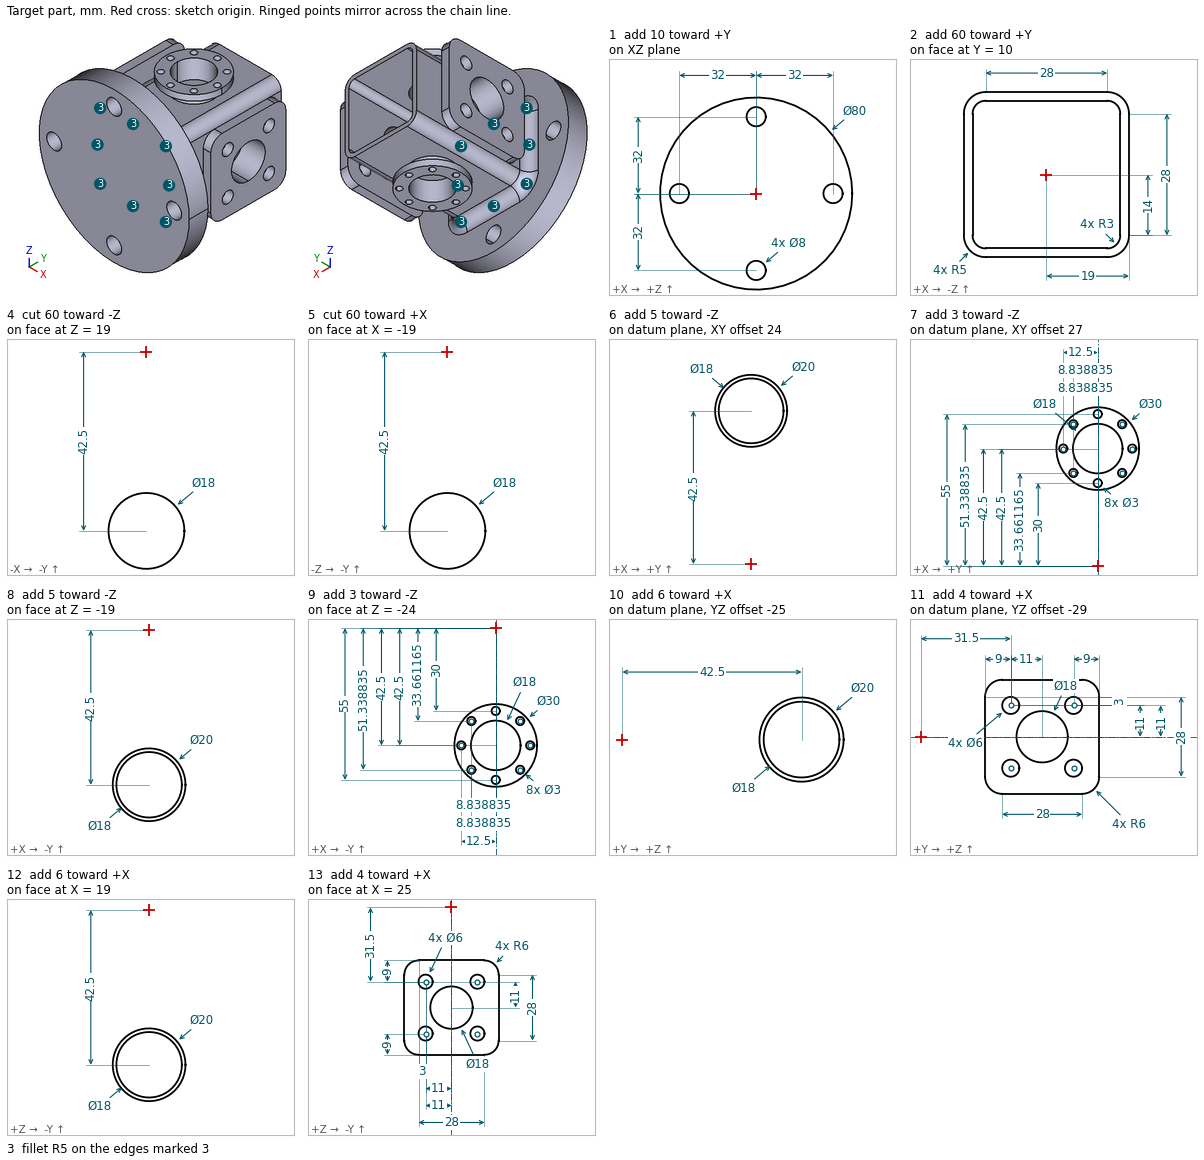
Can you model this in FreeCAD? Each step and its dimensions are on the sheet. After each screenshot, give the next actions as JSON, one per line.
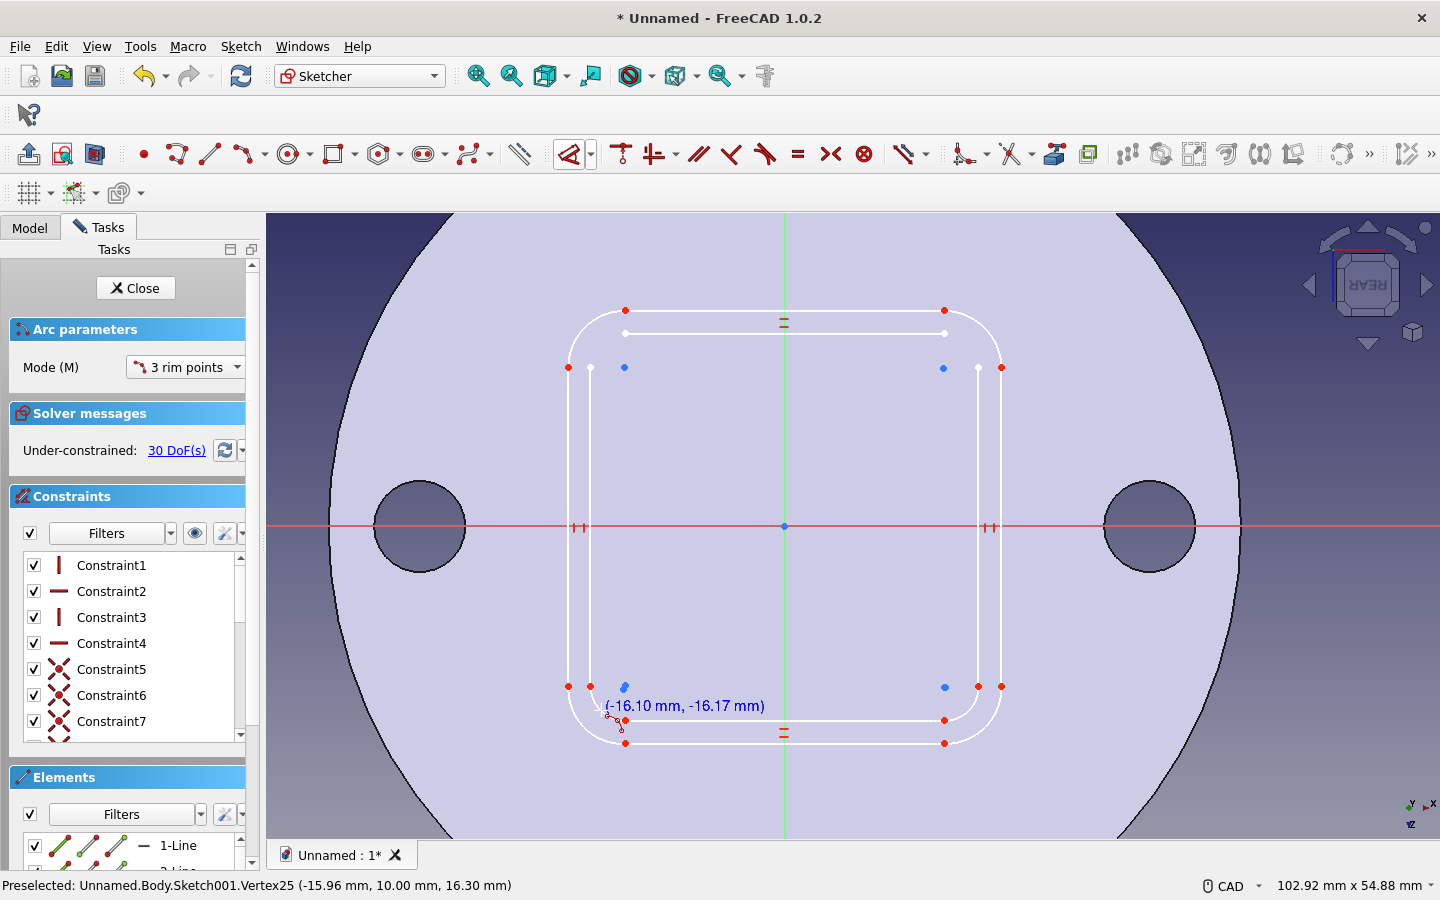
{"action": "left_click", "coordinate": [590, 368]}
{"action": "left_click", "coordinate": [625, 334]}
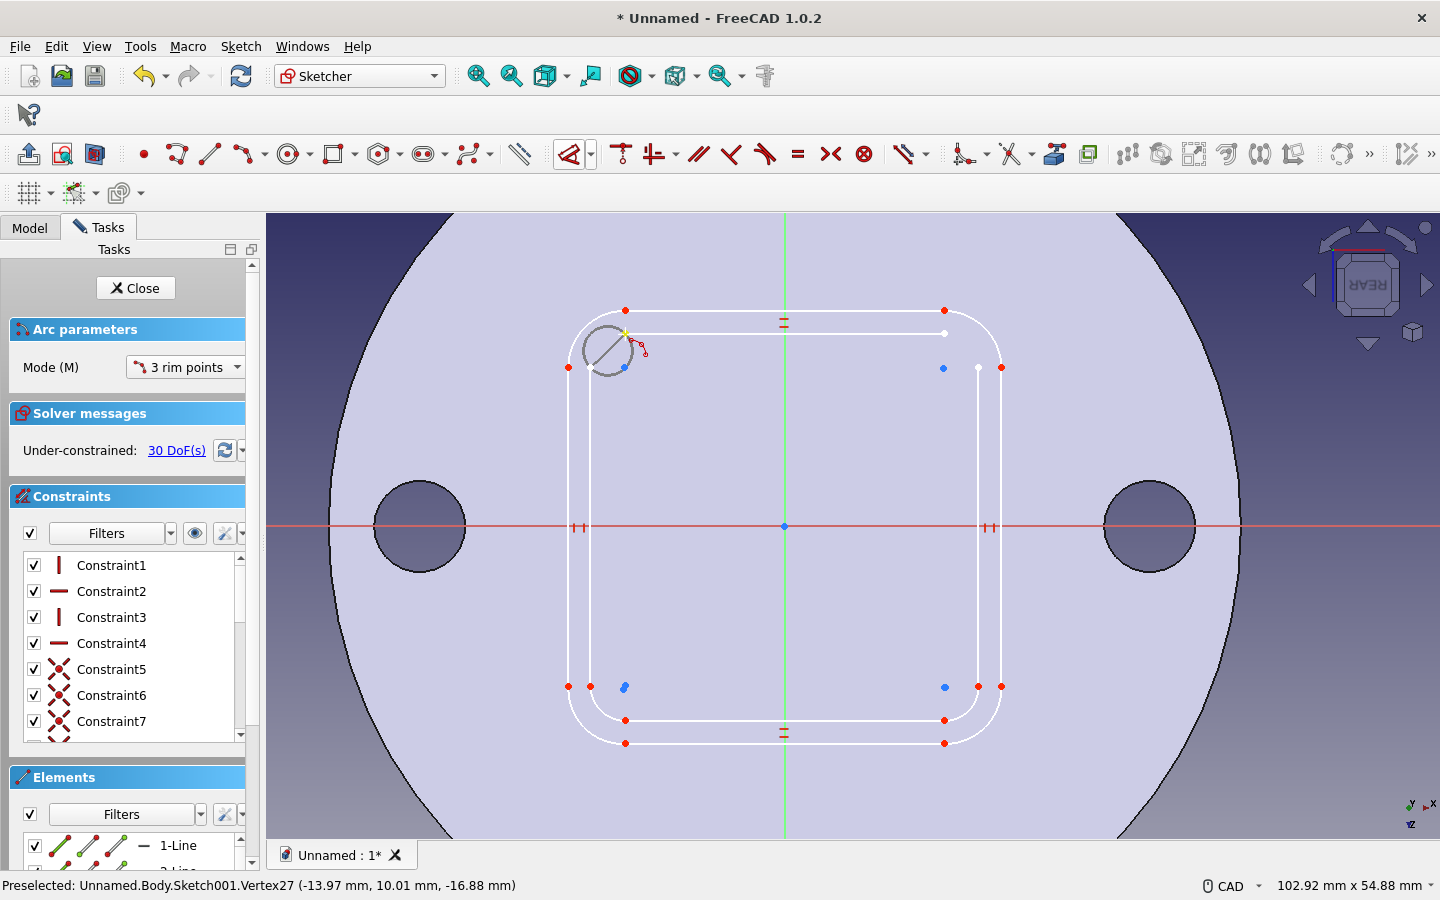
{"action": "scroll", "coordinate": [601, 343], "scroll_direction": "up", "scroll_amount": 3}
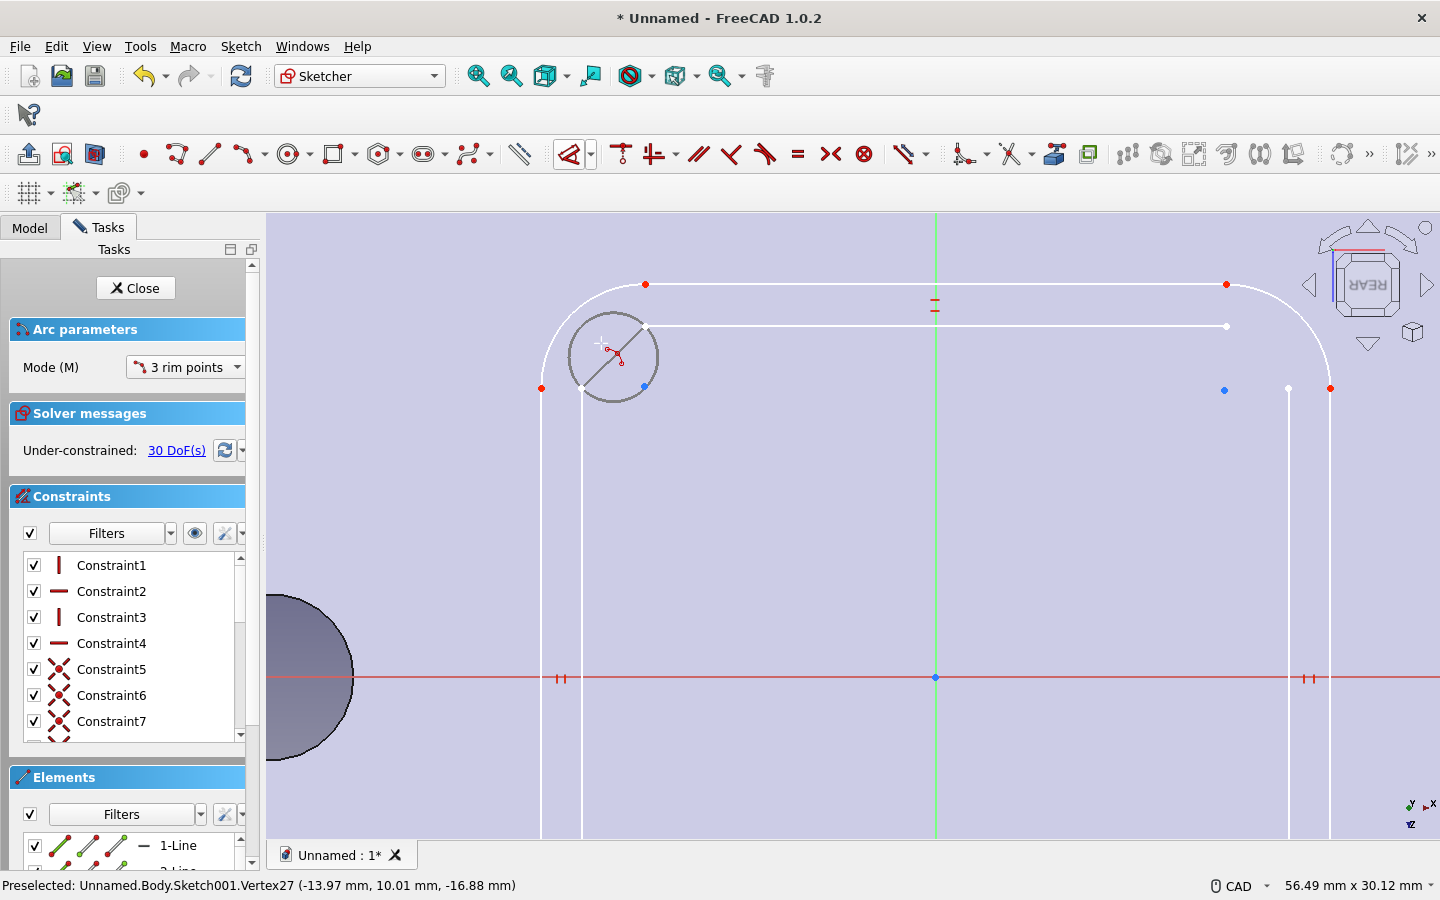
{"action": "left_click", "coordinate": [601, 342]}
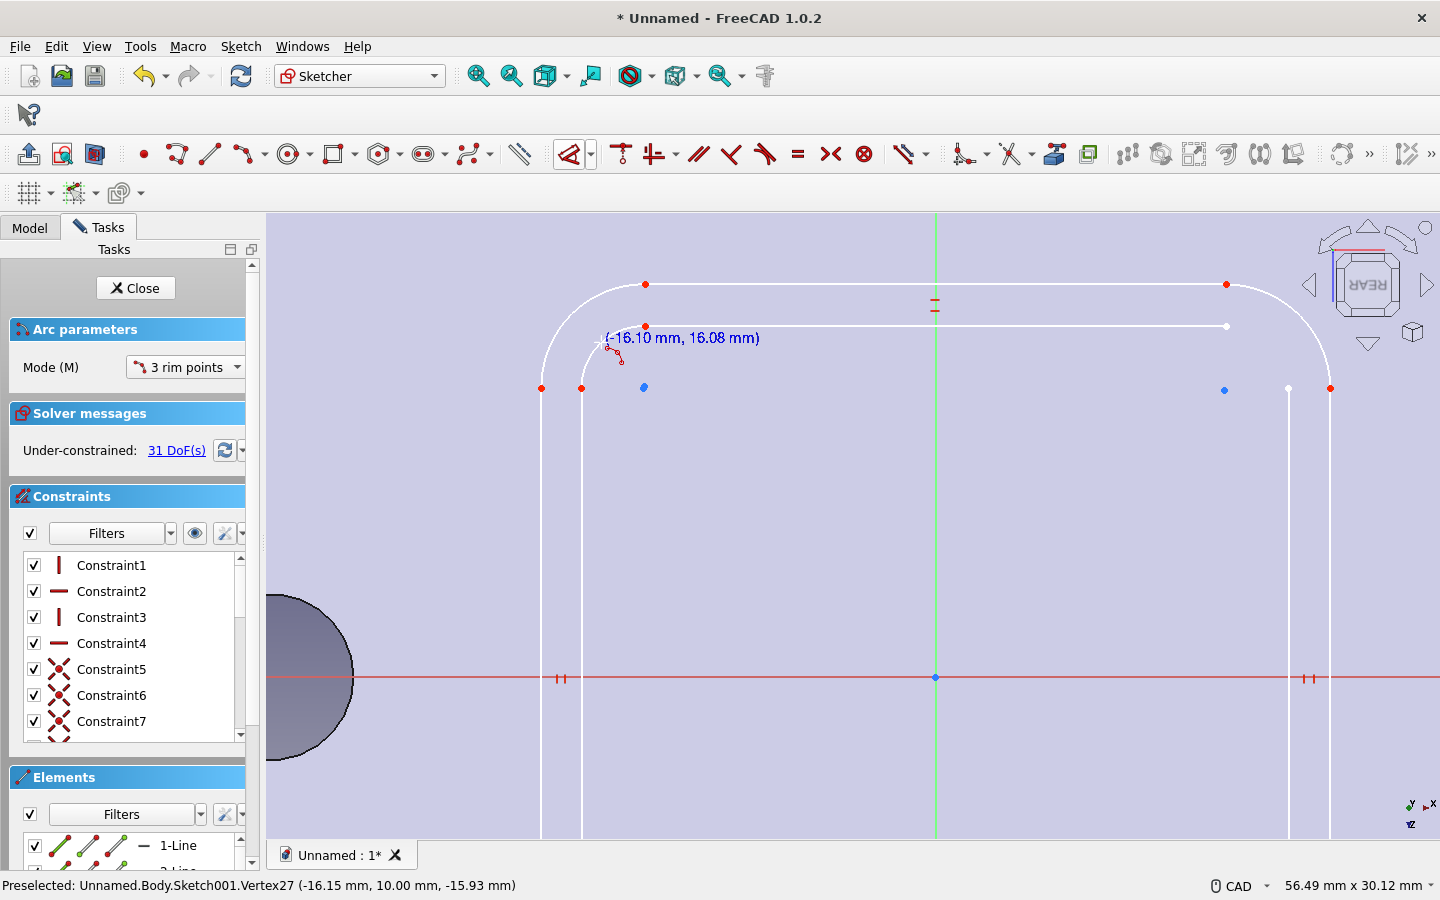
{"action": "left_click", "coordinate": [1227, 326]}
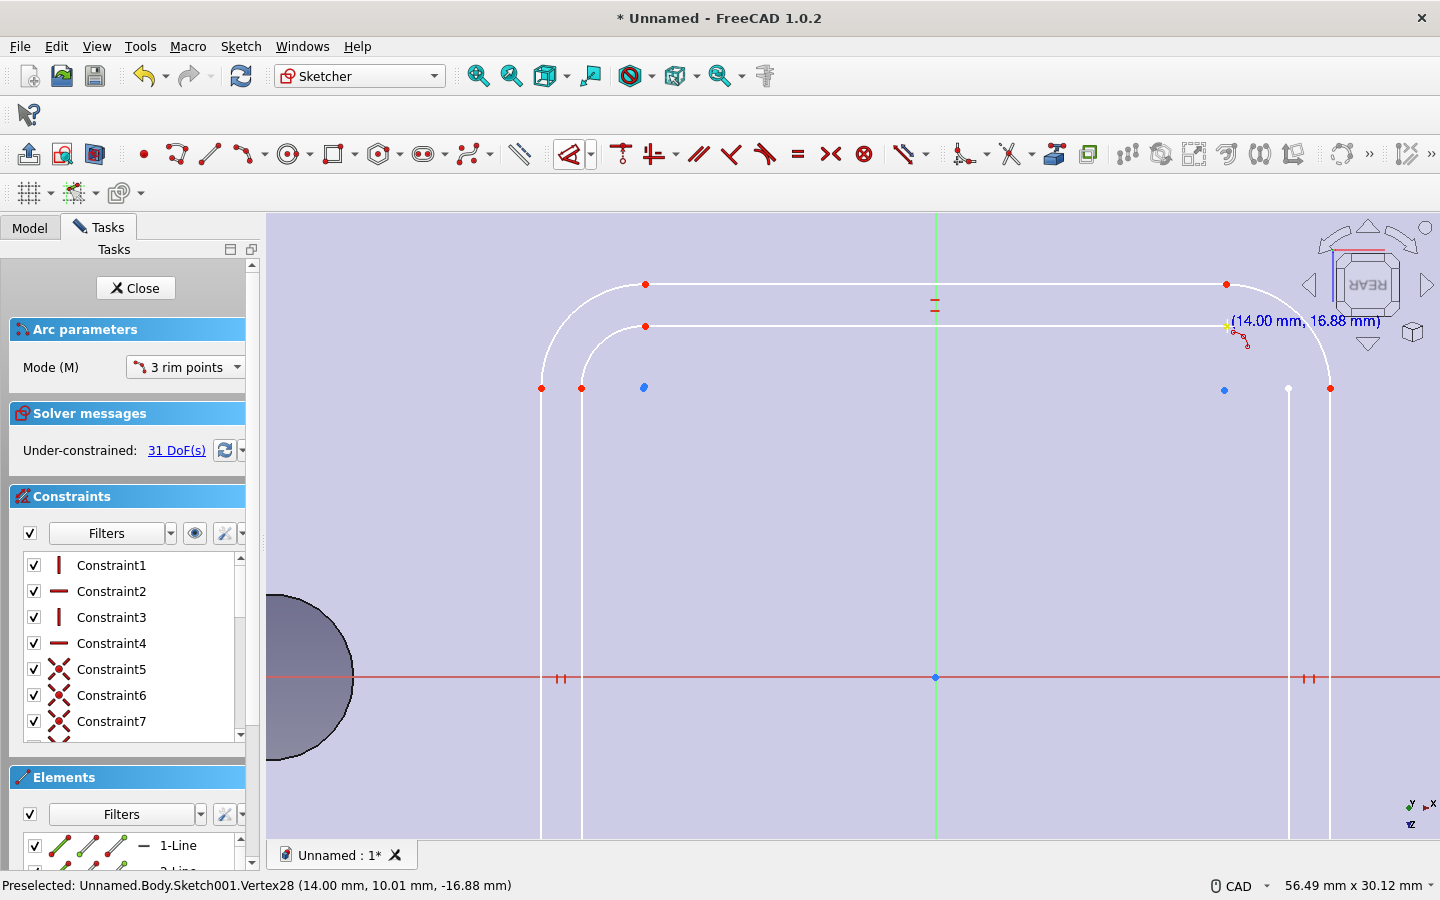
{"action": "scroll", "coordinate": [601, 342], "scroll_direction": "down", "scroll_amount": 3}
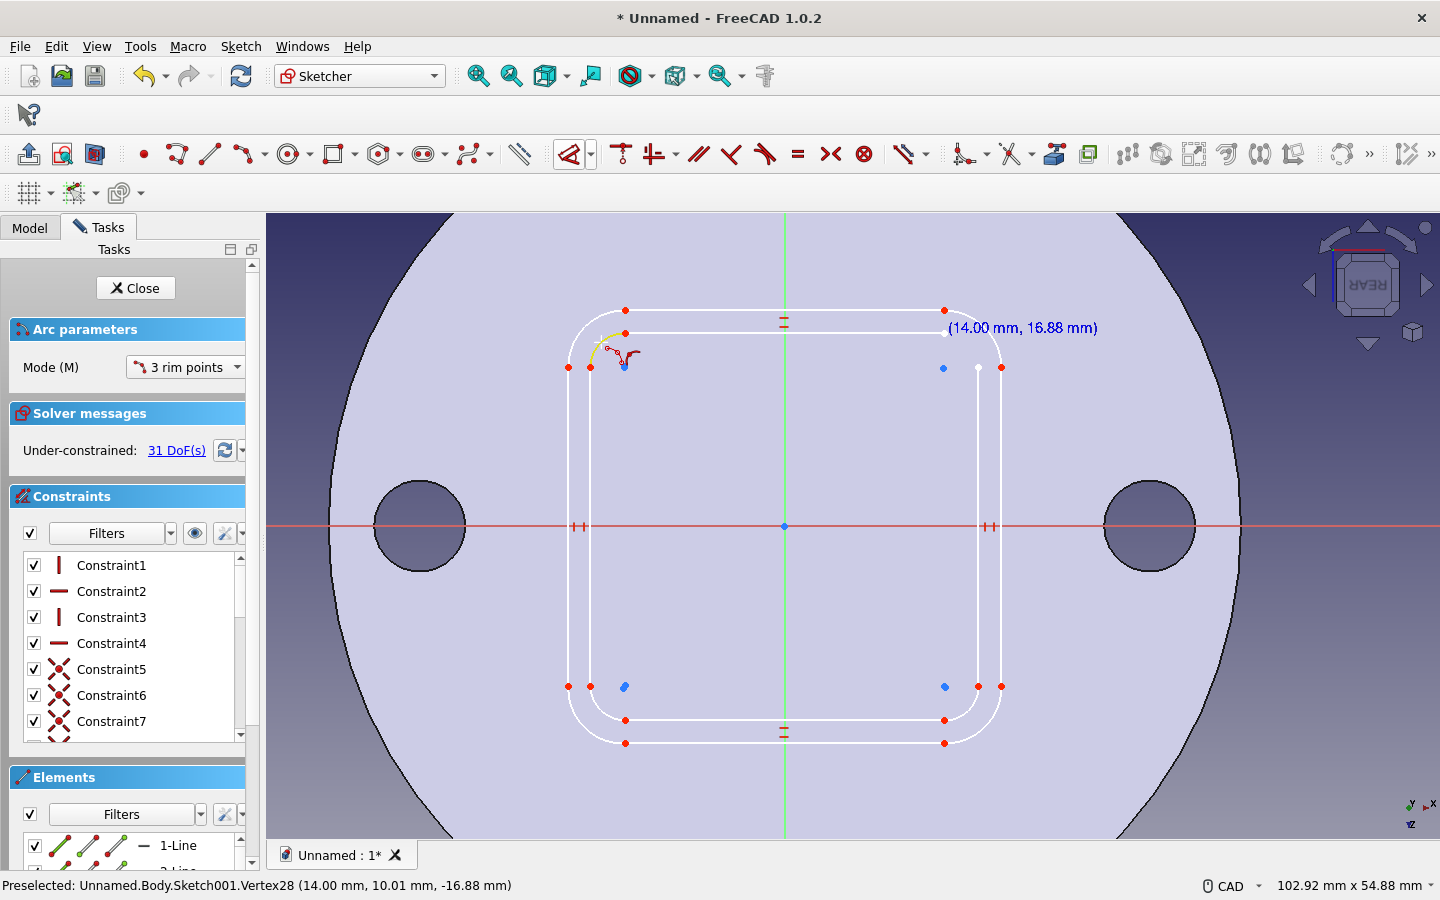
{"action": "left_click", "coordinate": [978, 367]}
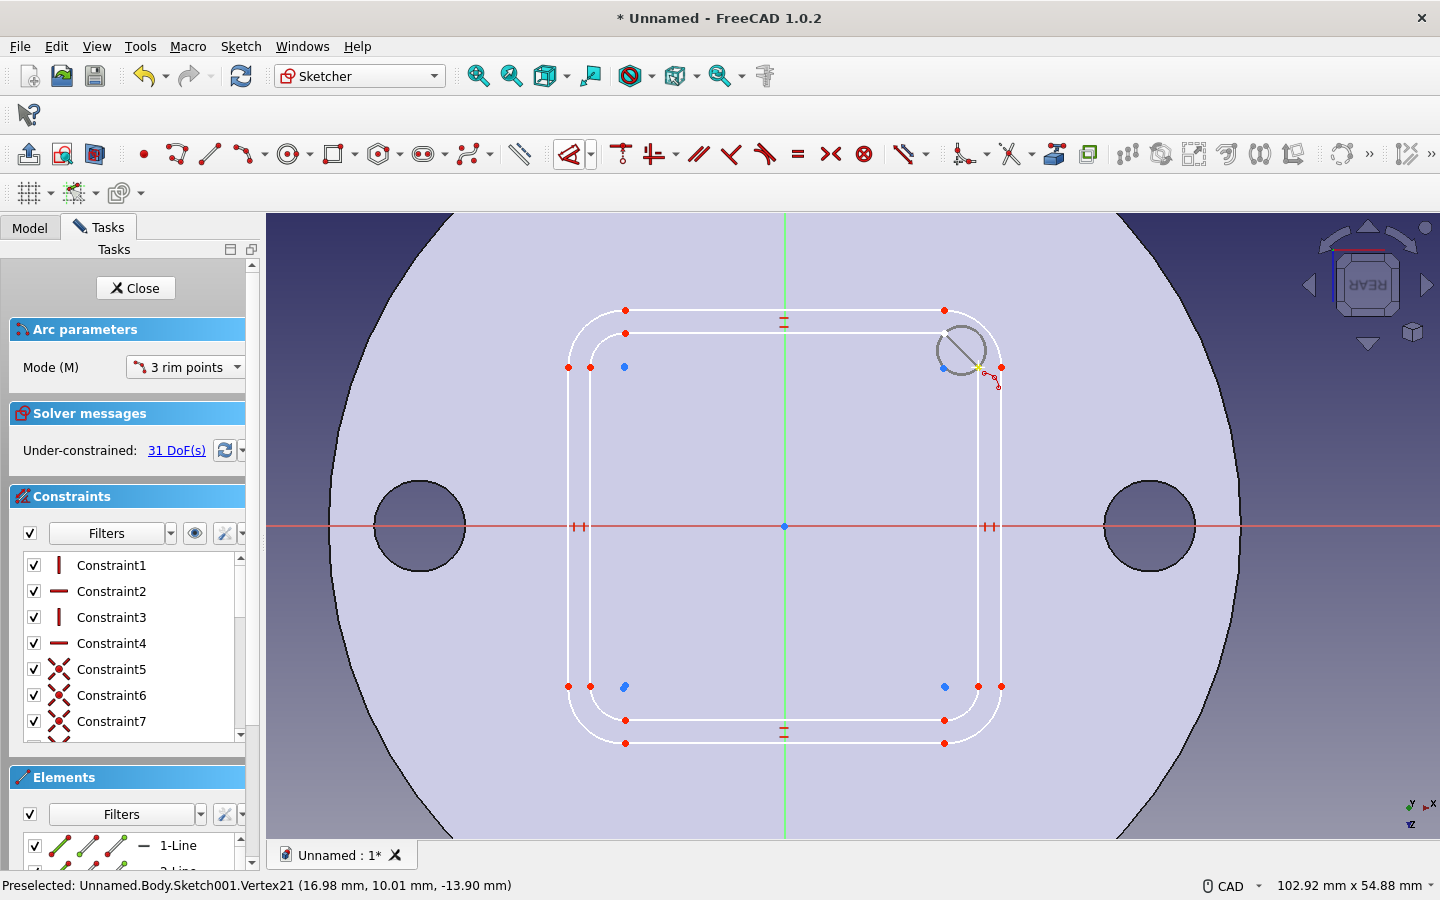
{"action": "scroll", "coordinate": [969, 342], "scroll_direction": "up", "scroll_amount": 3}